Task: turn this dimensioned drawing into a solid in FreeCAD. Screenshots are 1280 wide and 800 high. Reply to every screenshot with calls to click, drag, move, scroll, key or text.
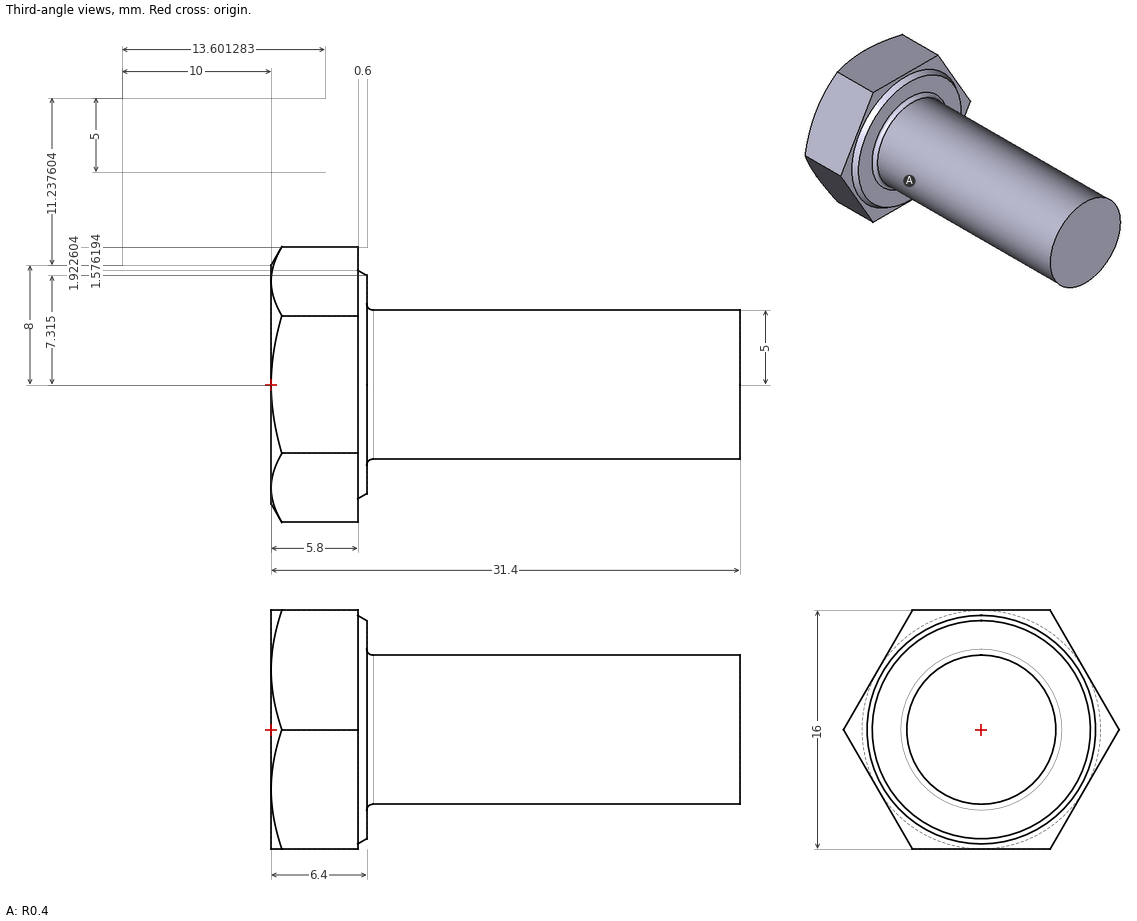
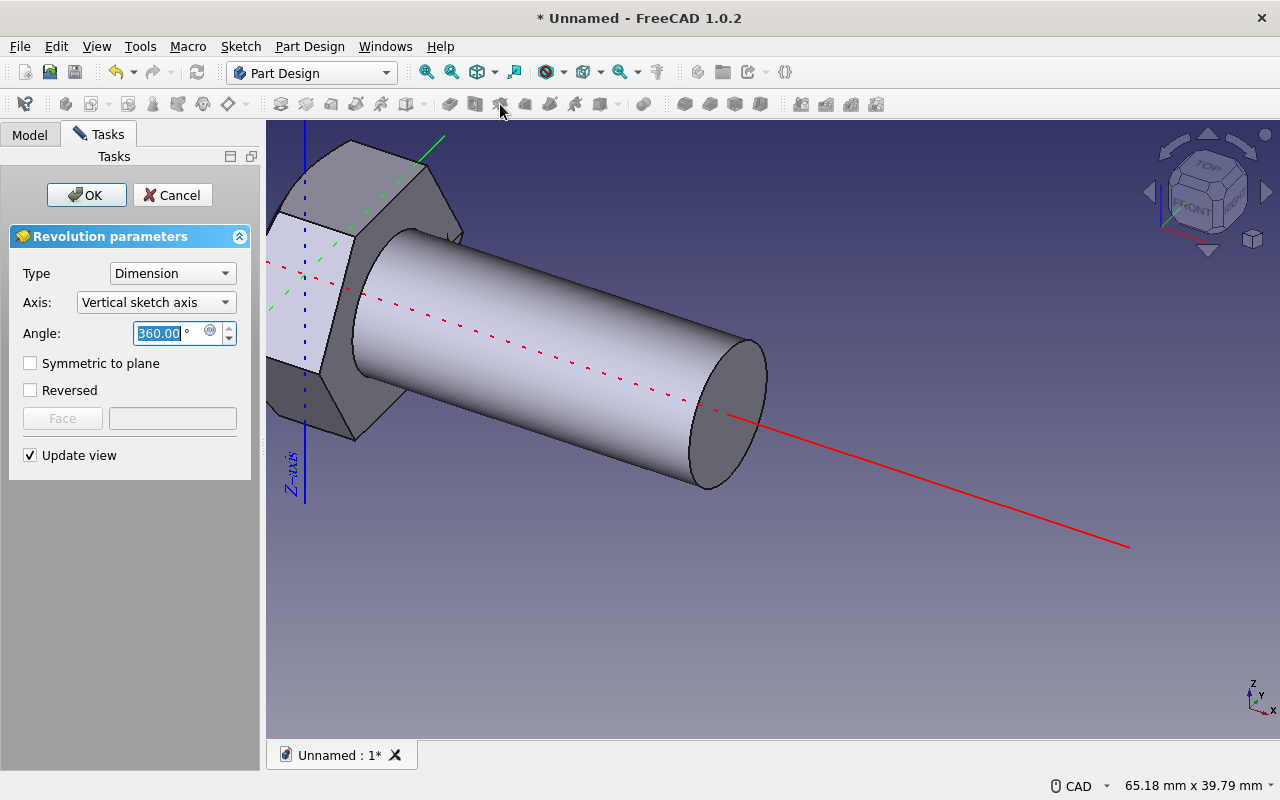
click(157, 302)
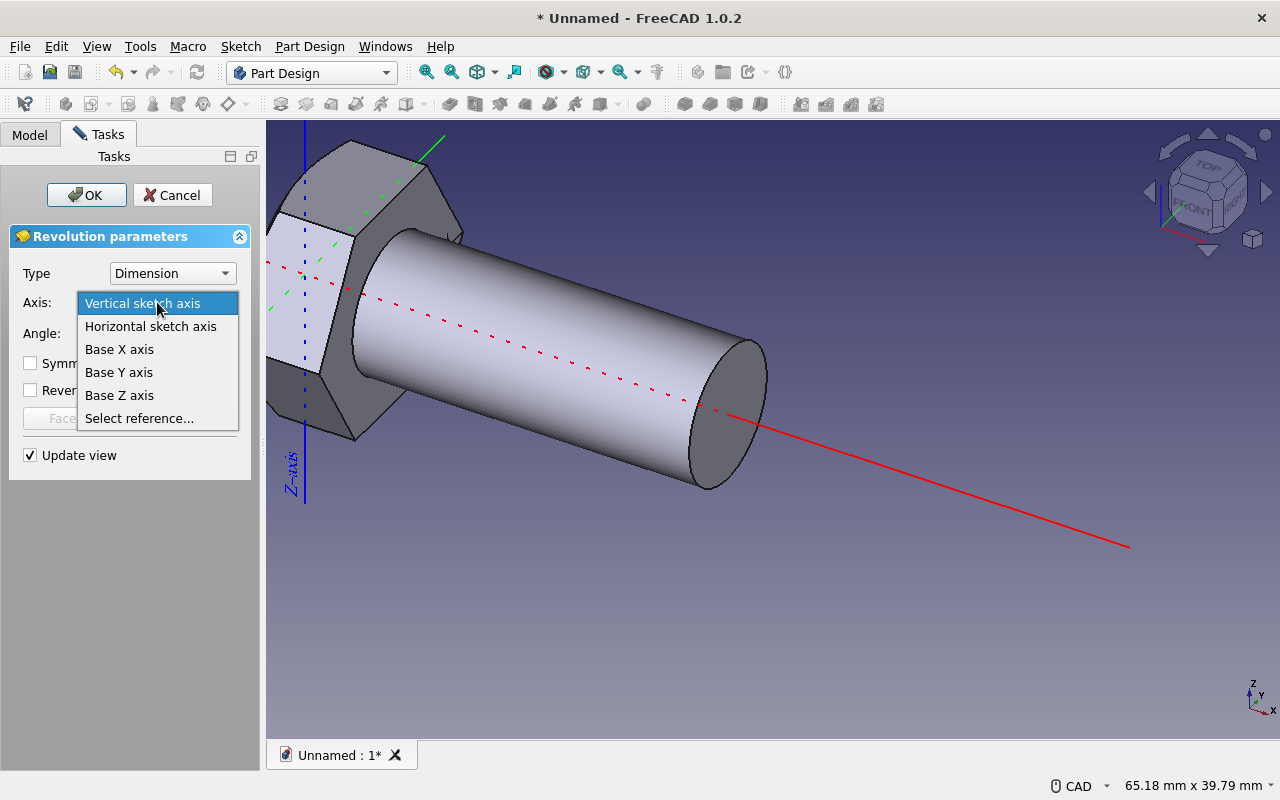
click(156, 326)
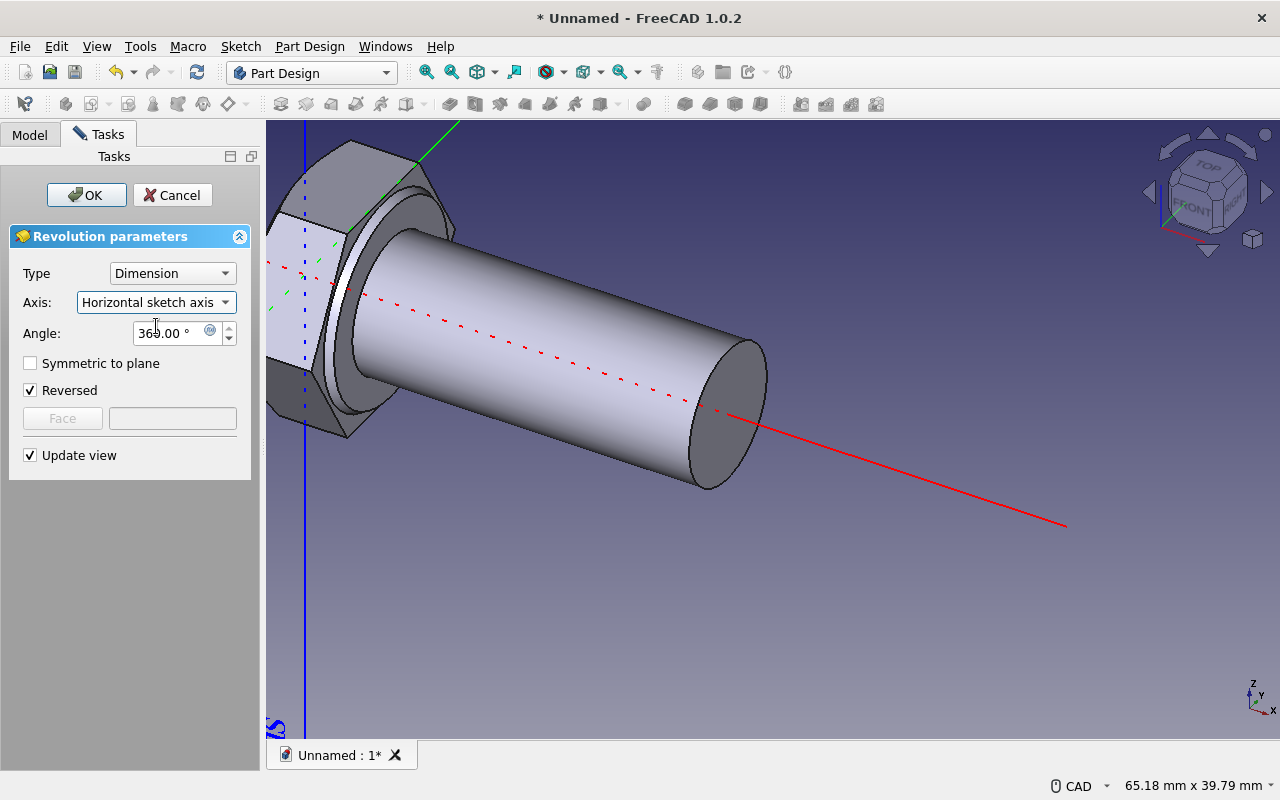
click(87, 195)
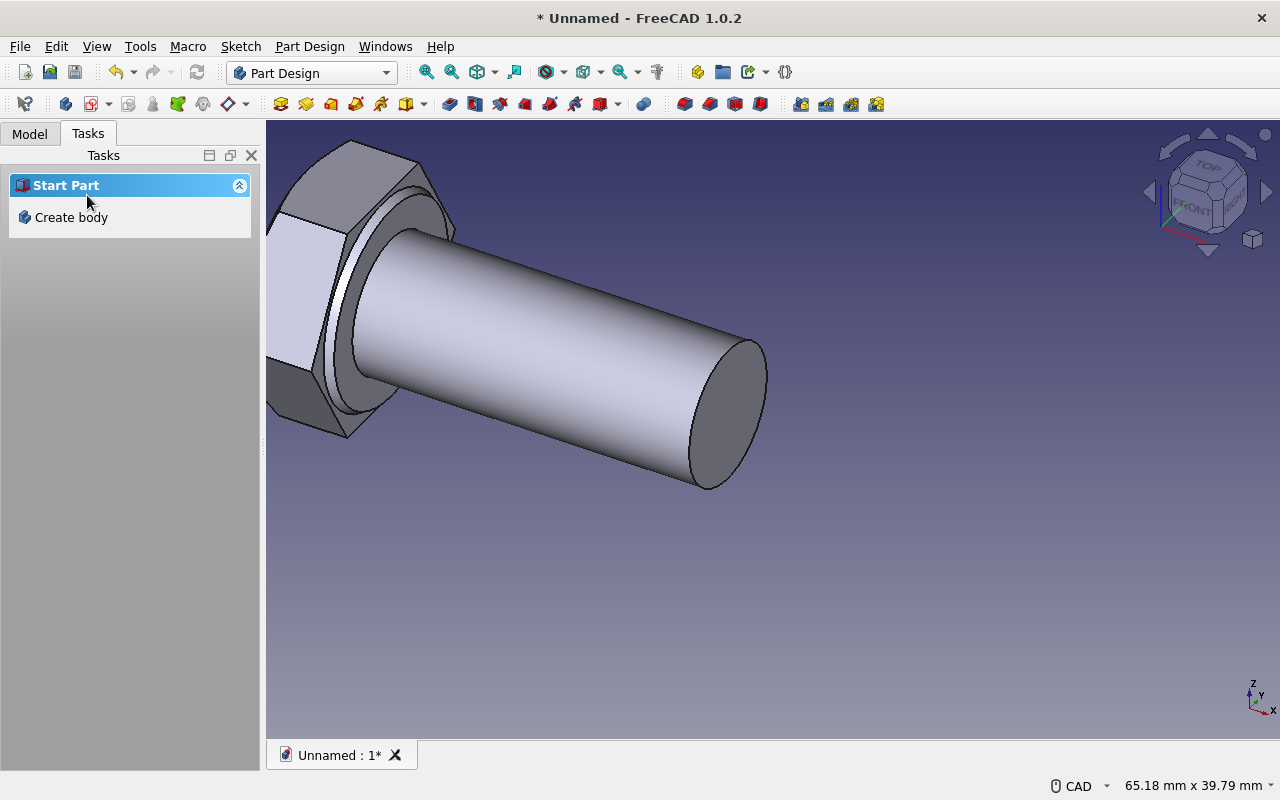
key(v)
key(f)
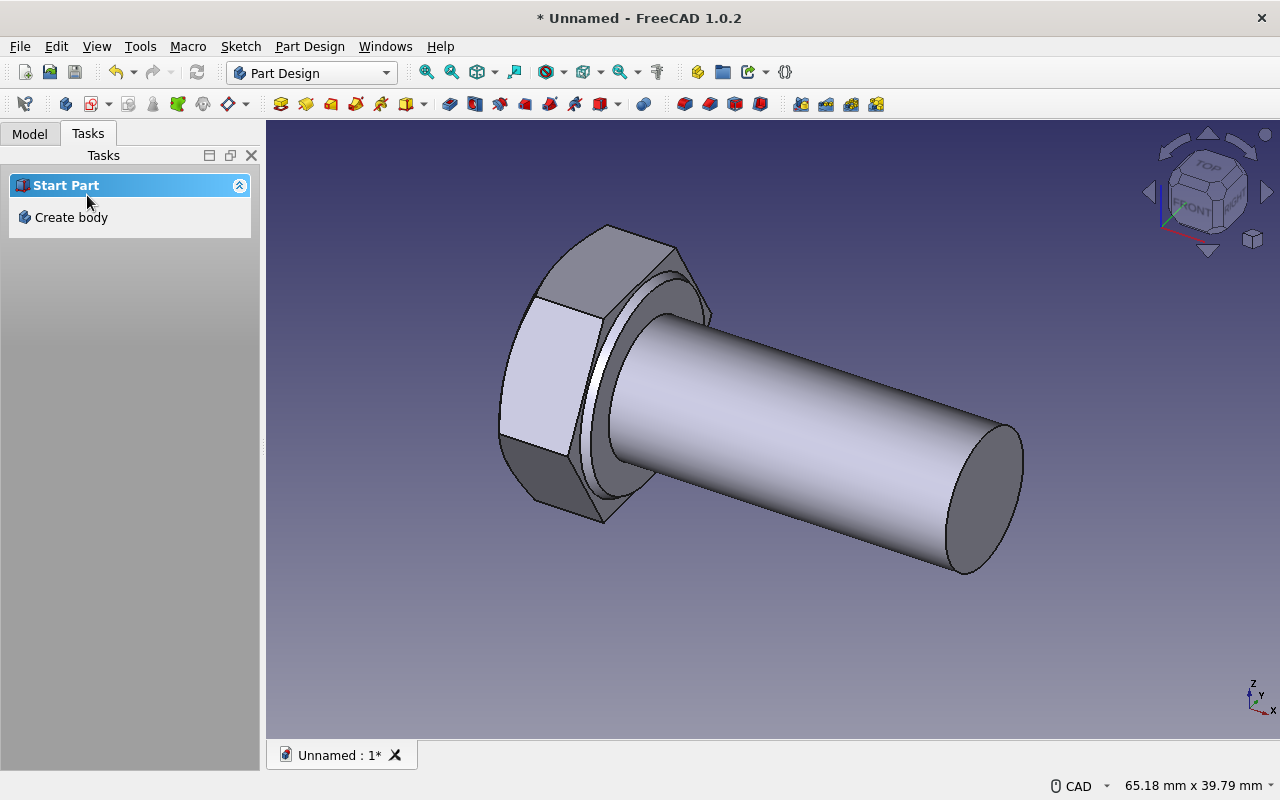
key(0)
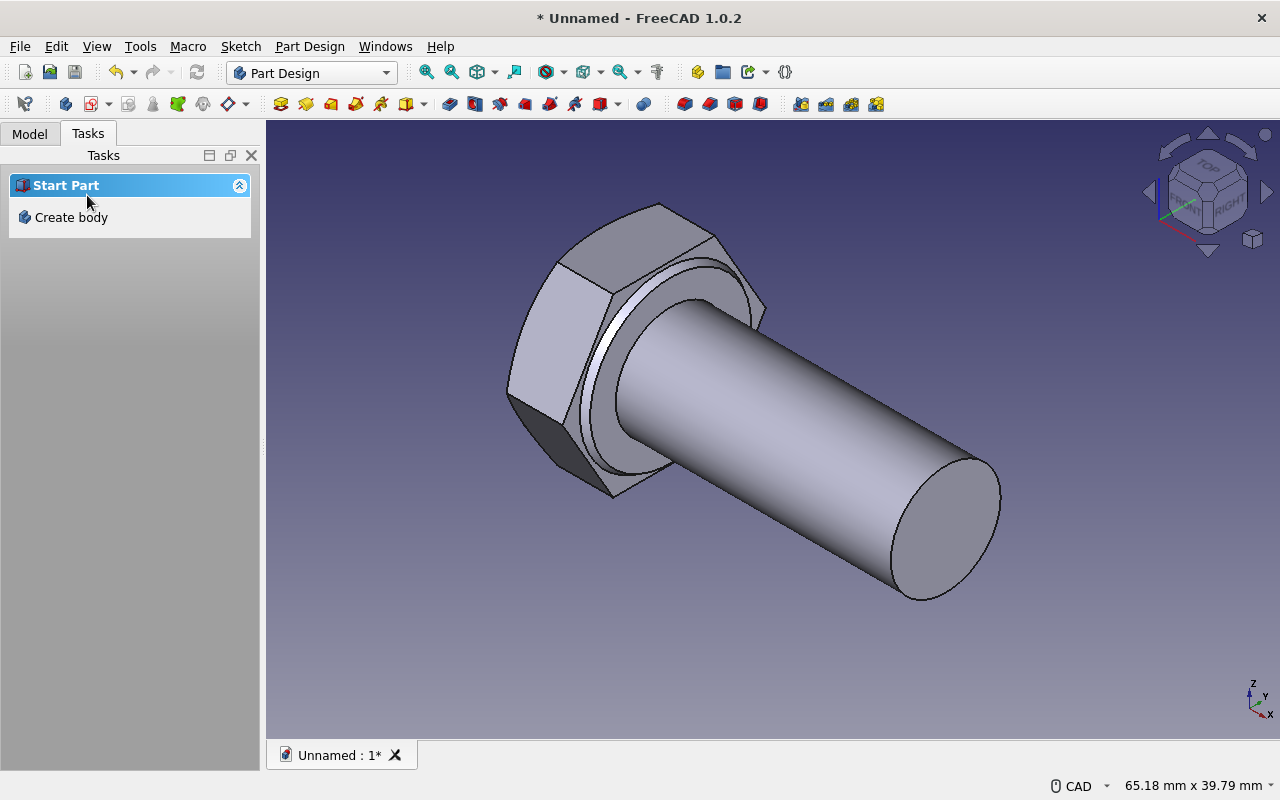
click(688, 299)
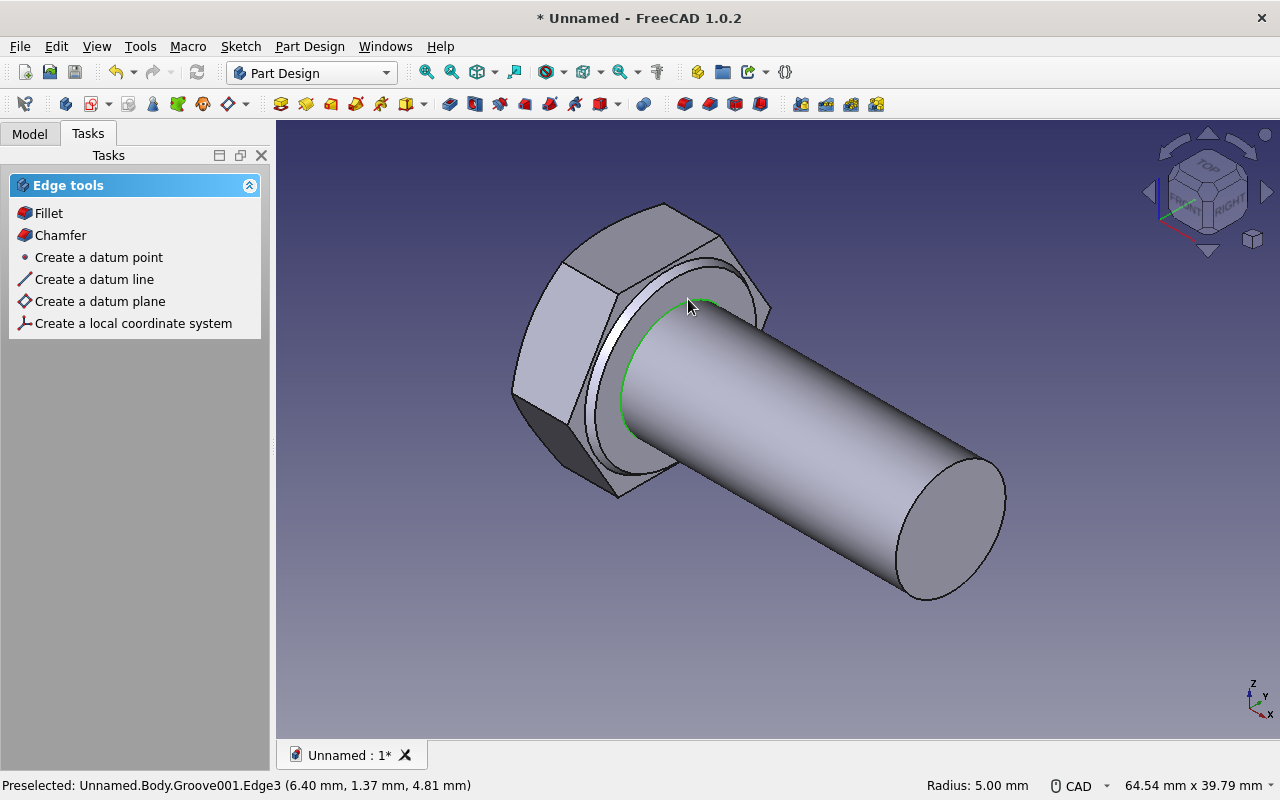
click(685, 104)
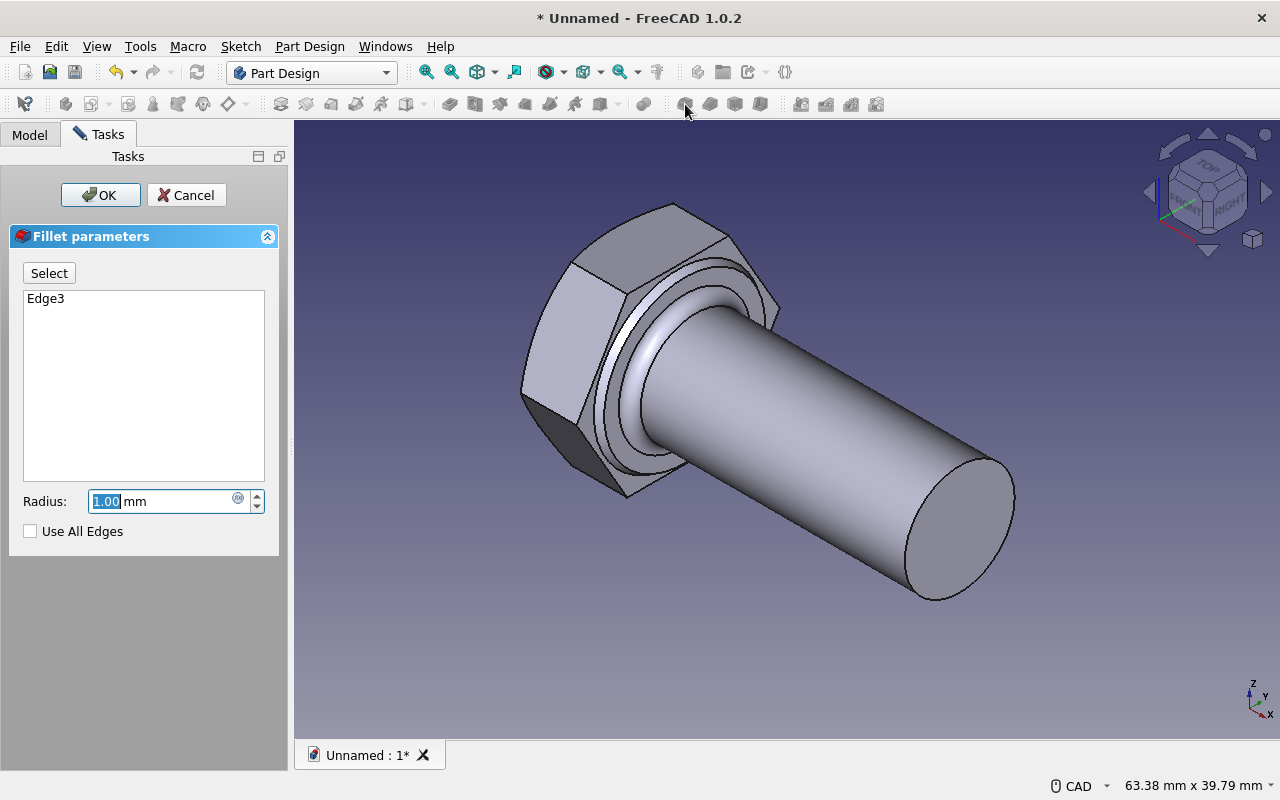
text(0.4)
key(Tab)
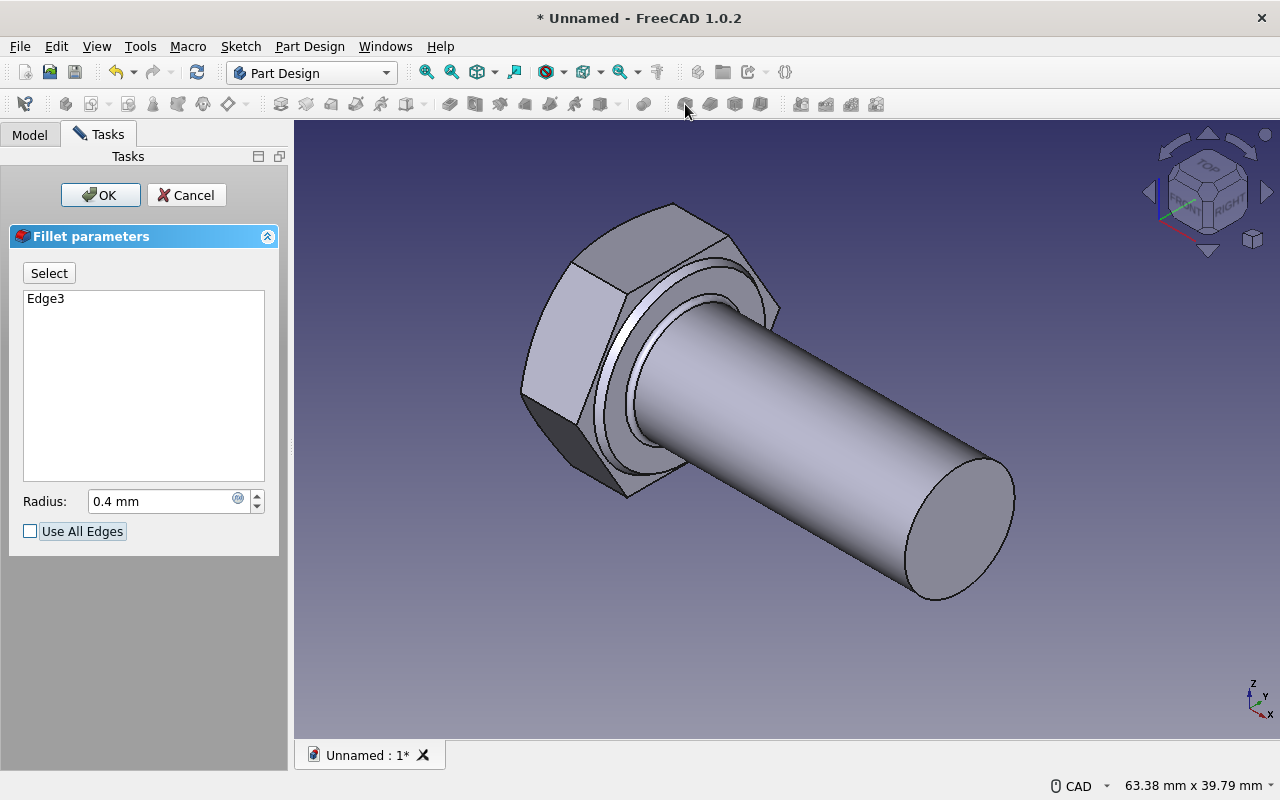
click(101, 195)